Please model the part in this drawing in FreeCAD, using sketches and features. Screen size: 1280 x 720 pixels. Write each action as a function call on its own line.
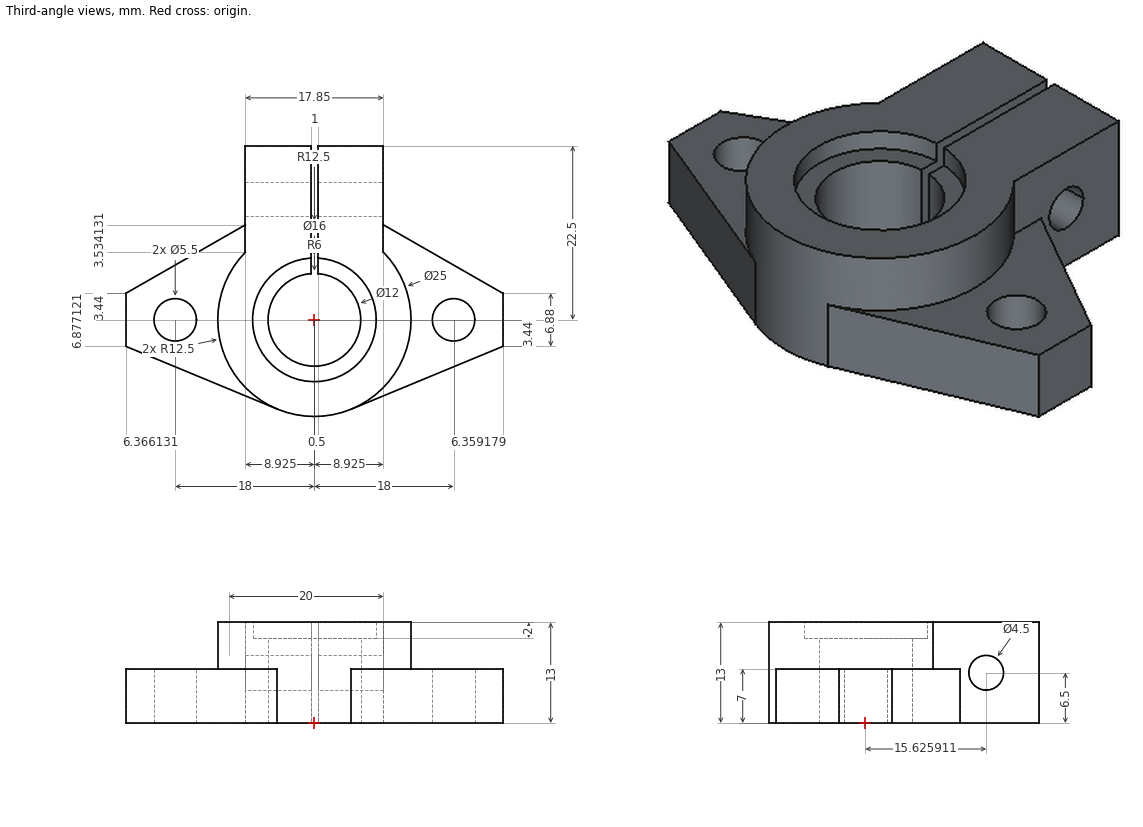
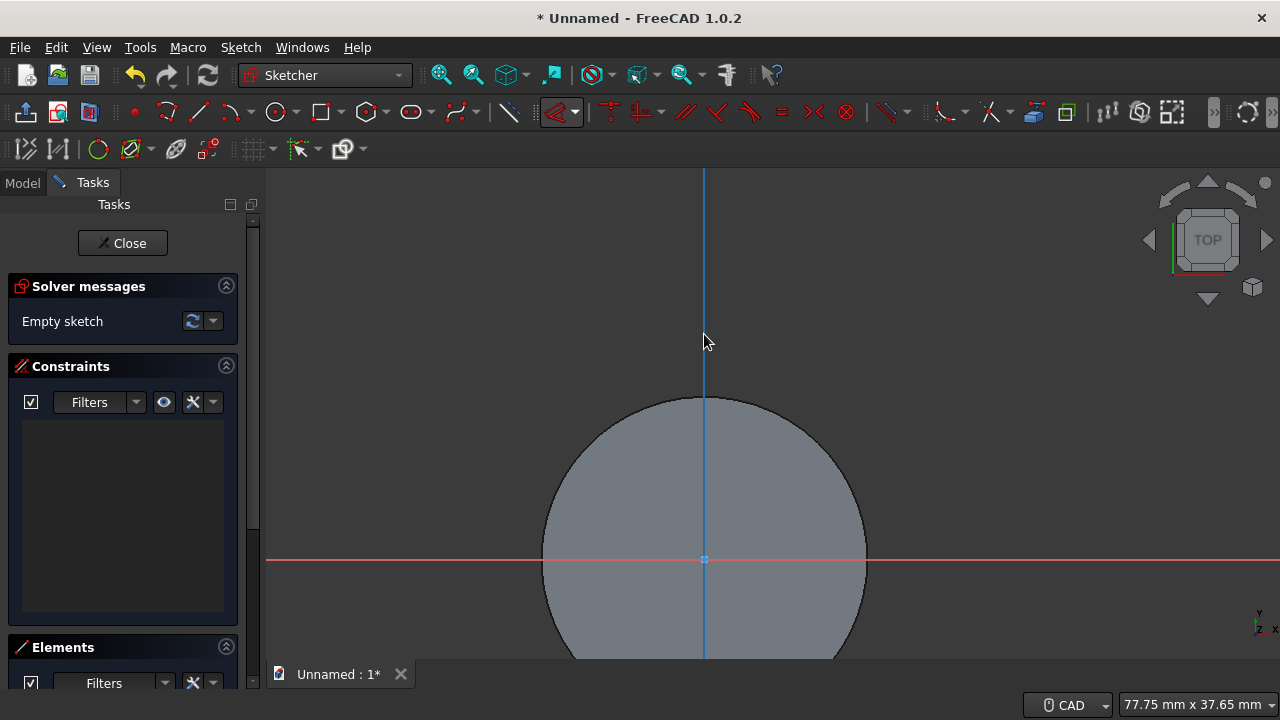
click(168, 112)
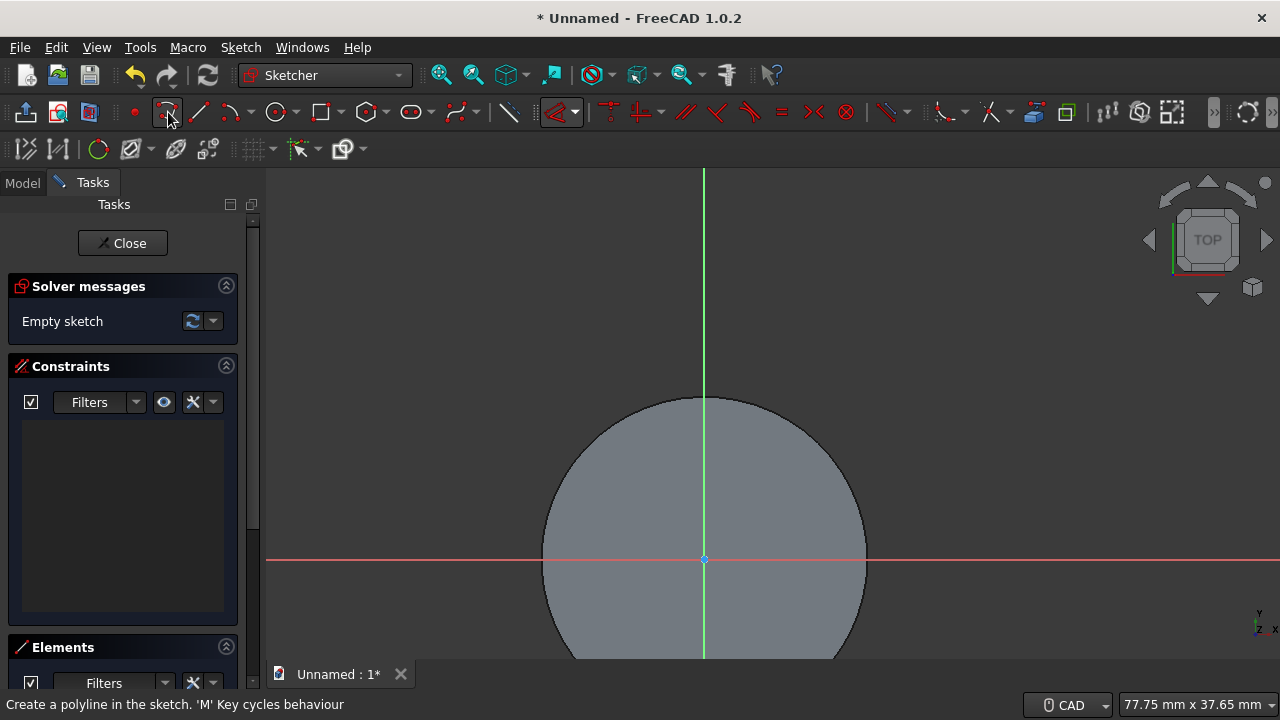
click(821, 446)
click(821, 266)
click(588, 266)
click(588, 446)
right_click(588, 446)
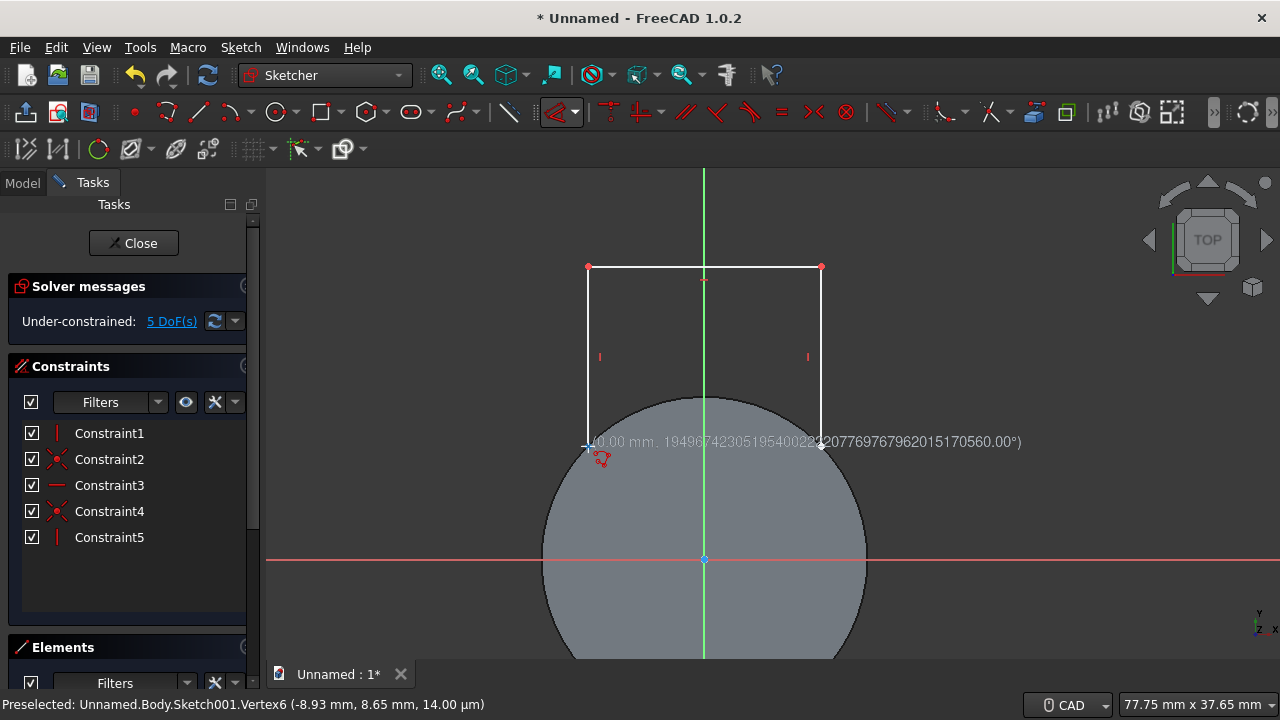
click(254, 112)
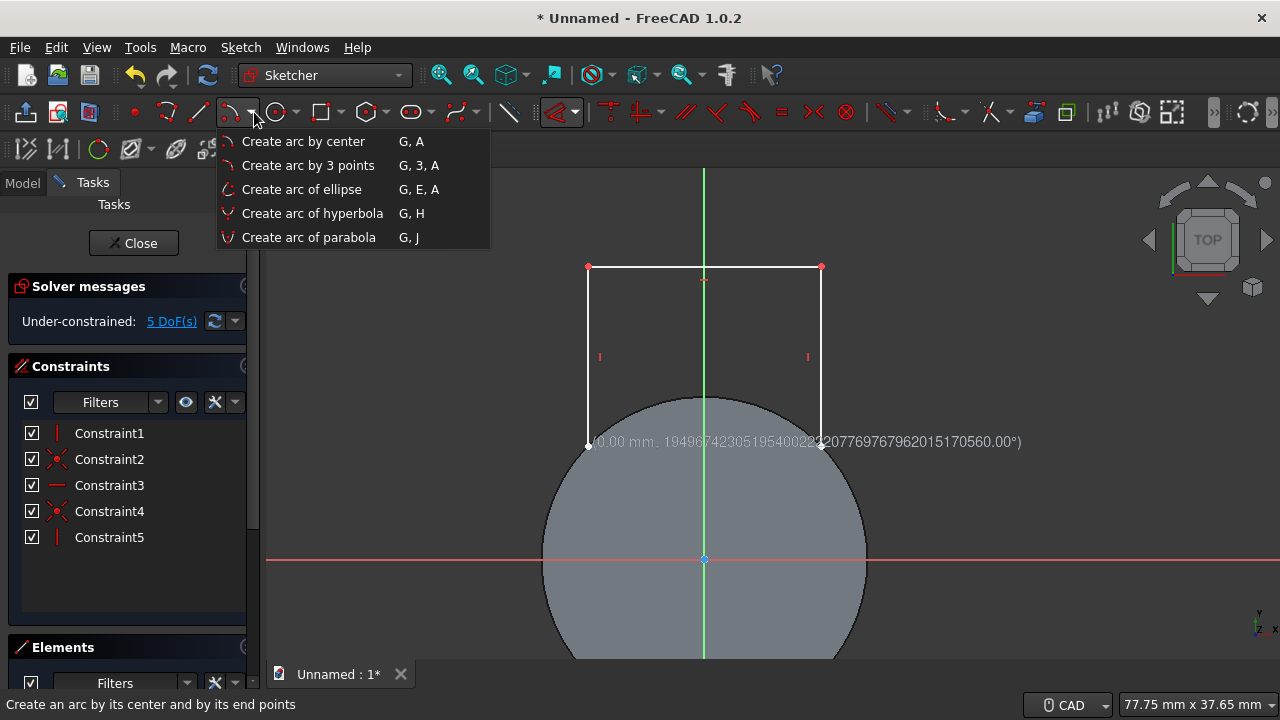
click(354, 165)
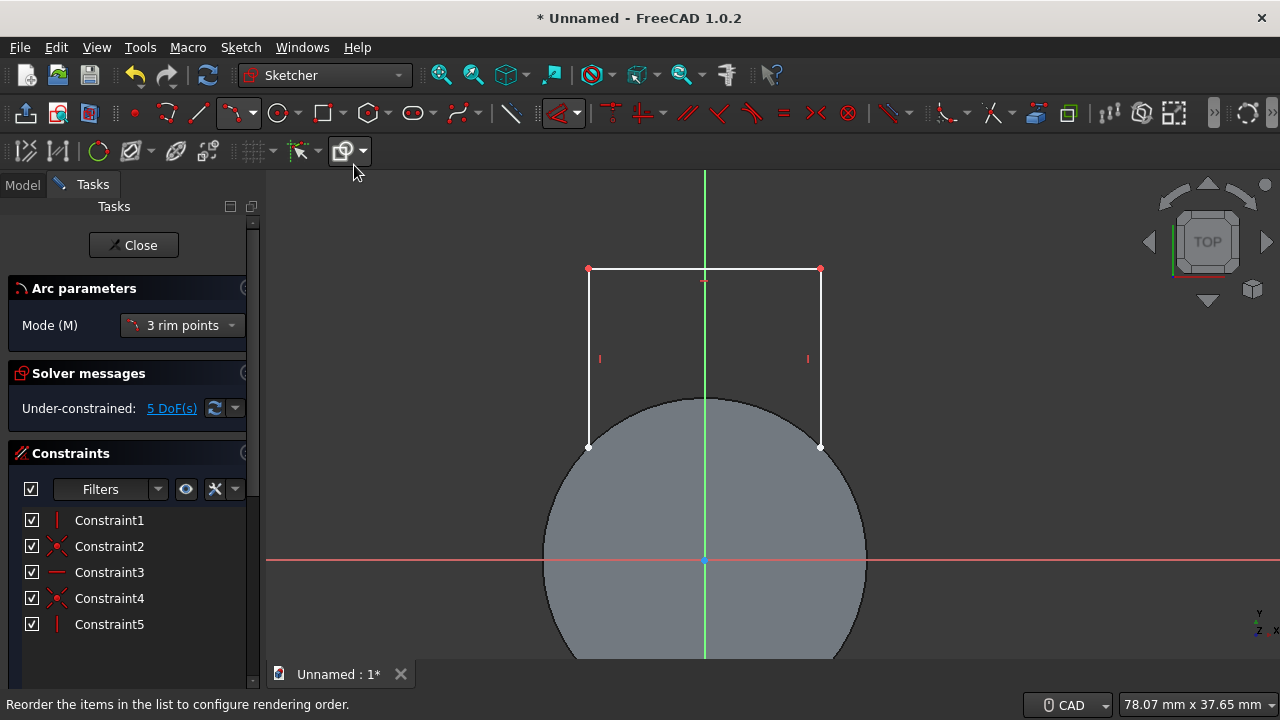
click(589, 448)
click(821, 448)
click(730, 400)
key(Escape)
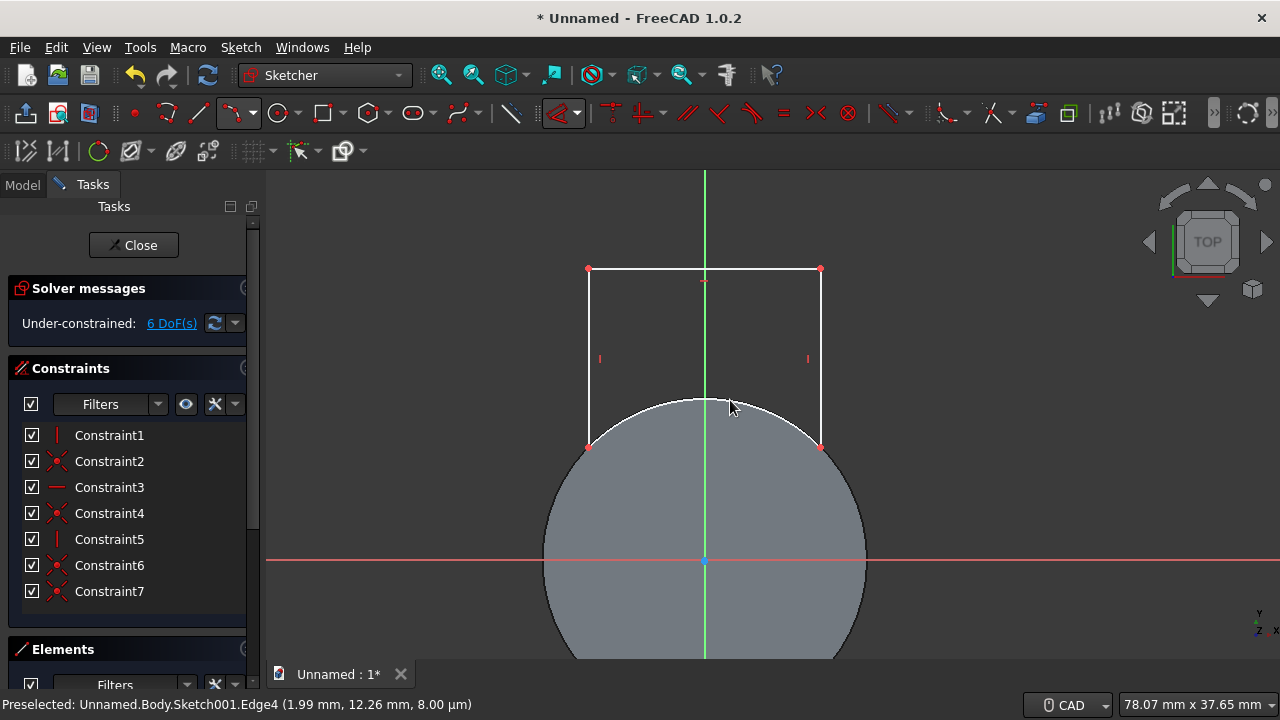
drag(695, 550, 715, 571)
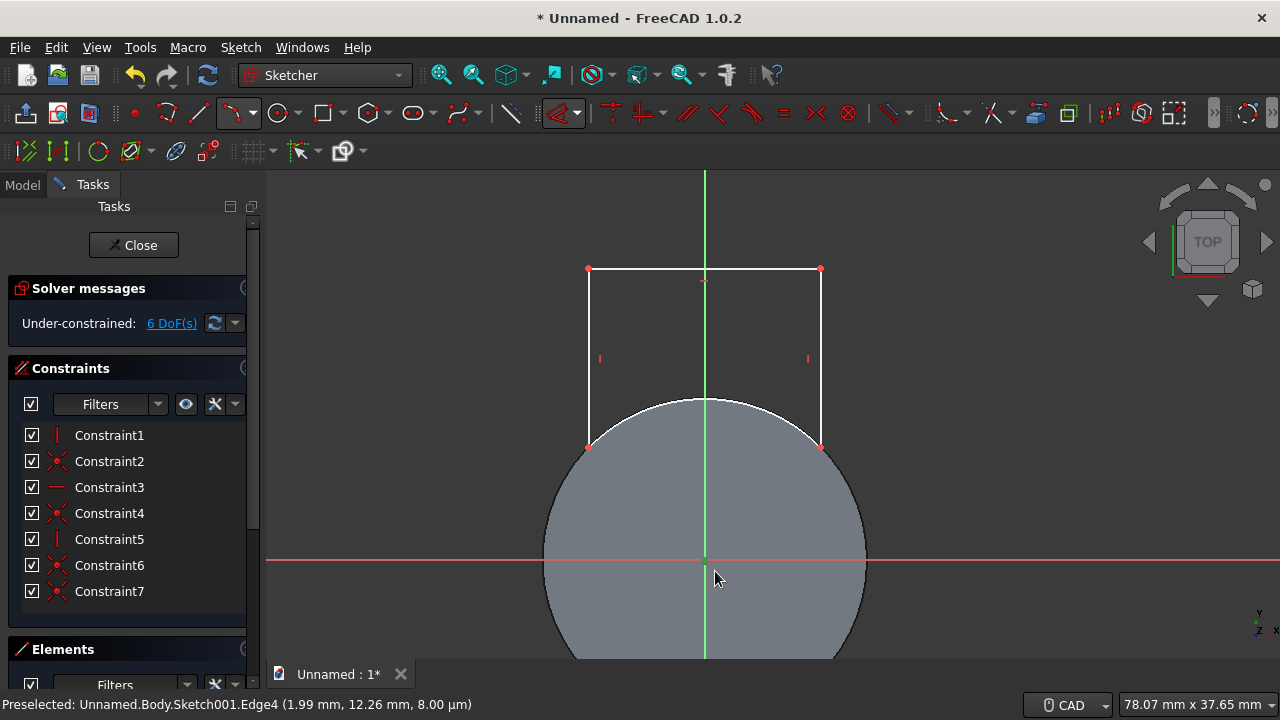
click(612, 114)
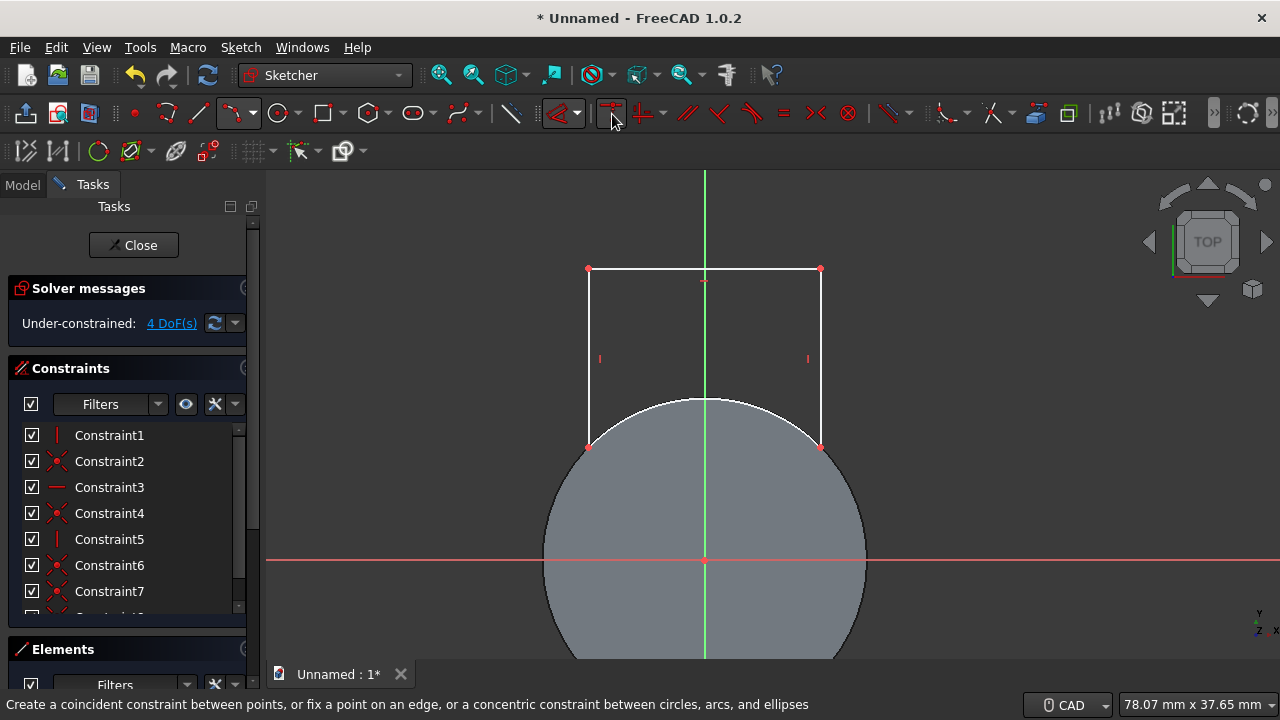
click(756, 407)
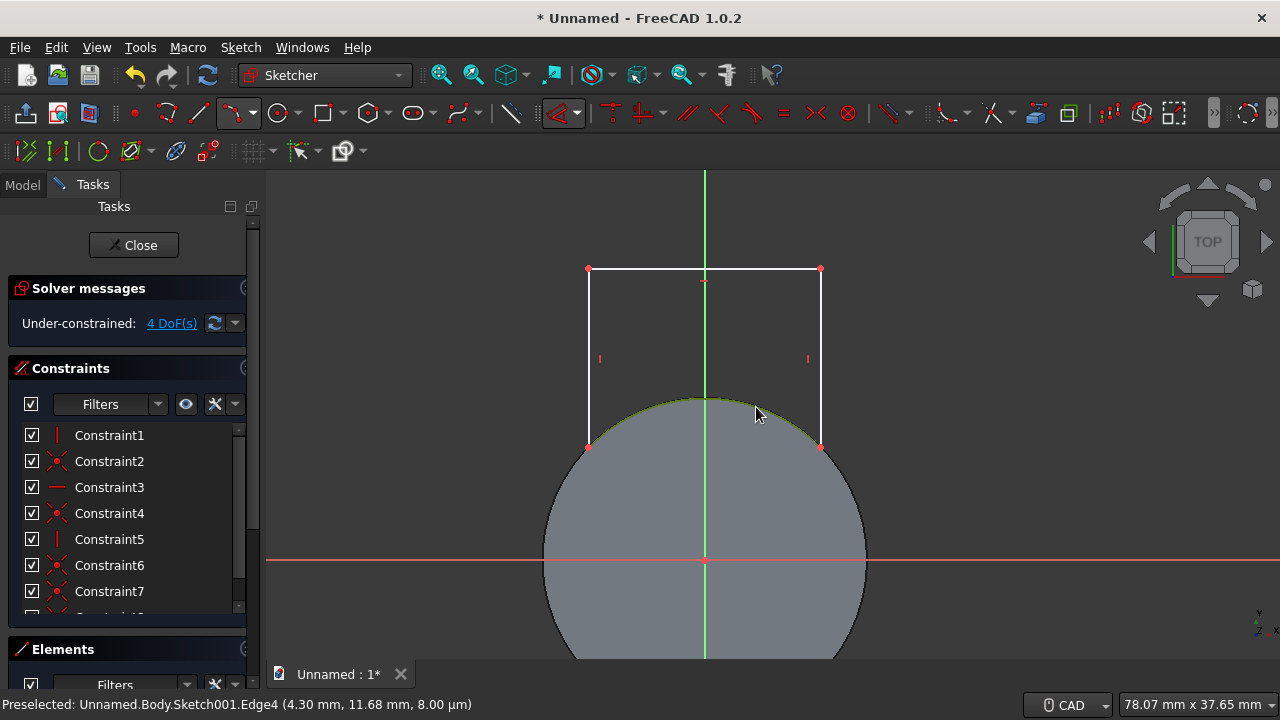
click(580, 114)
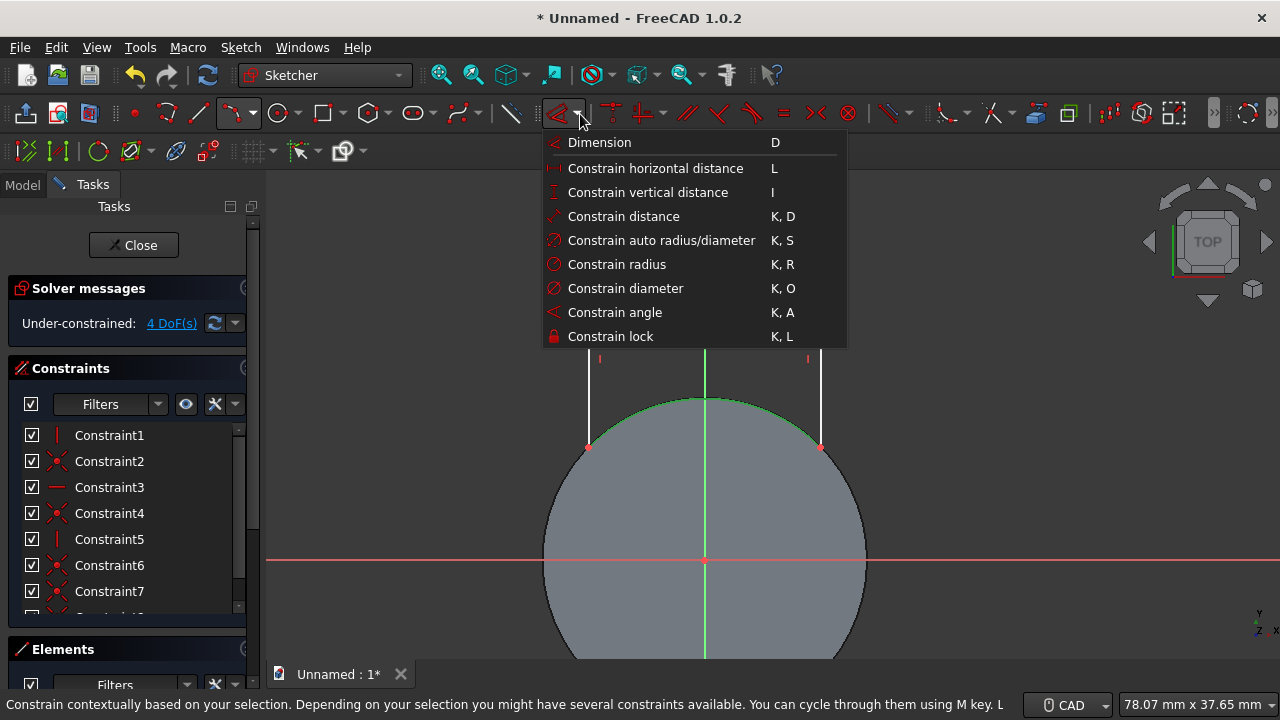
click(695, 264)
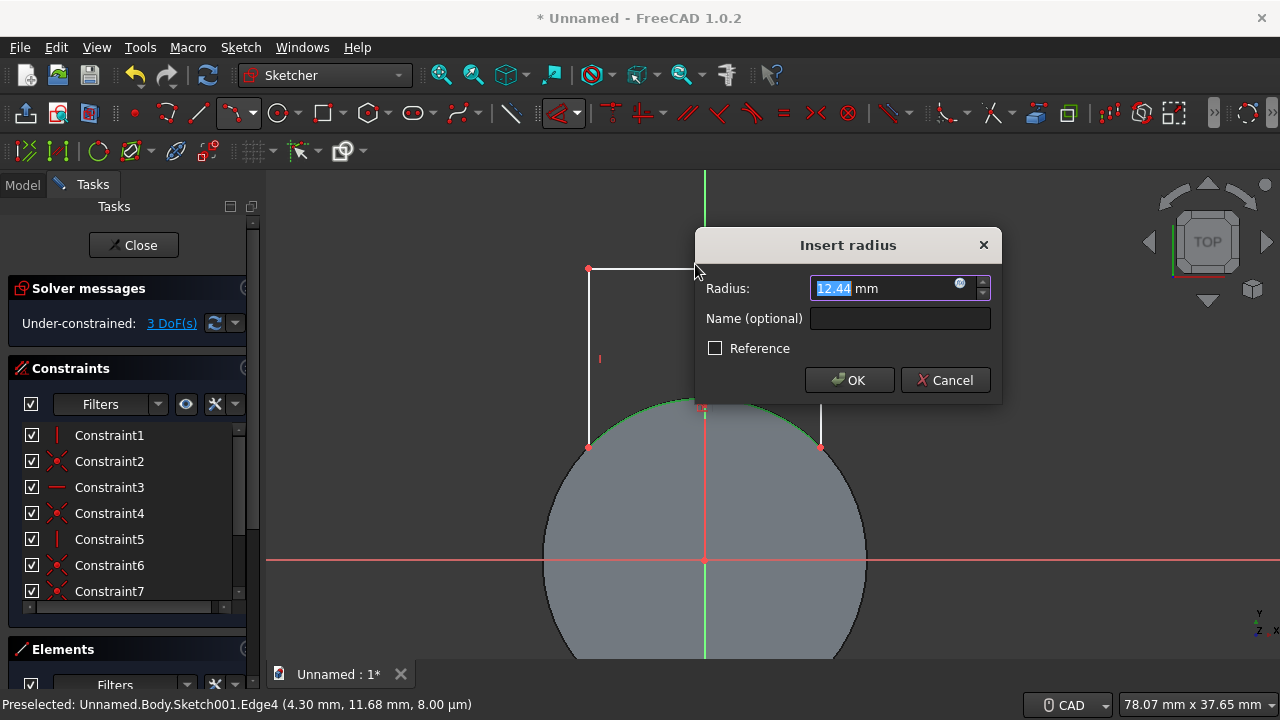
text(12.5)
key(Return)